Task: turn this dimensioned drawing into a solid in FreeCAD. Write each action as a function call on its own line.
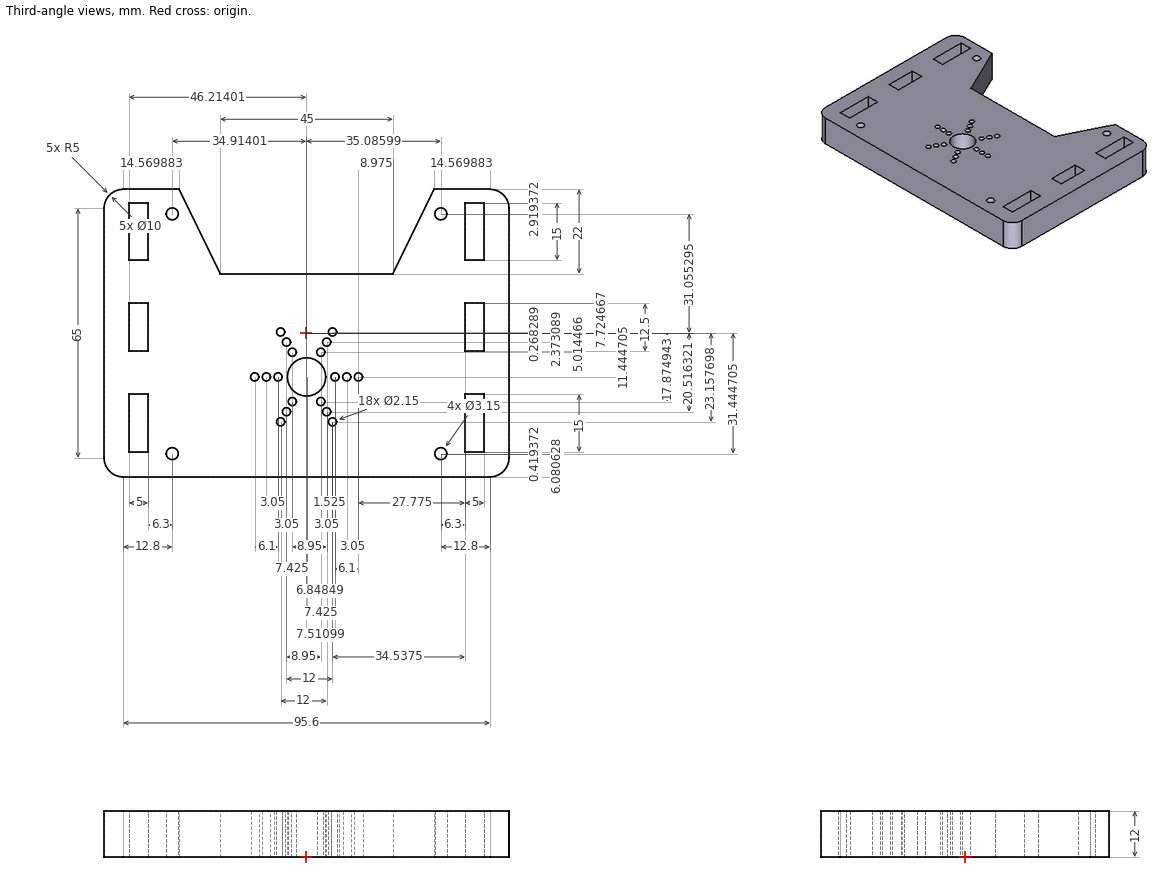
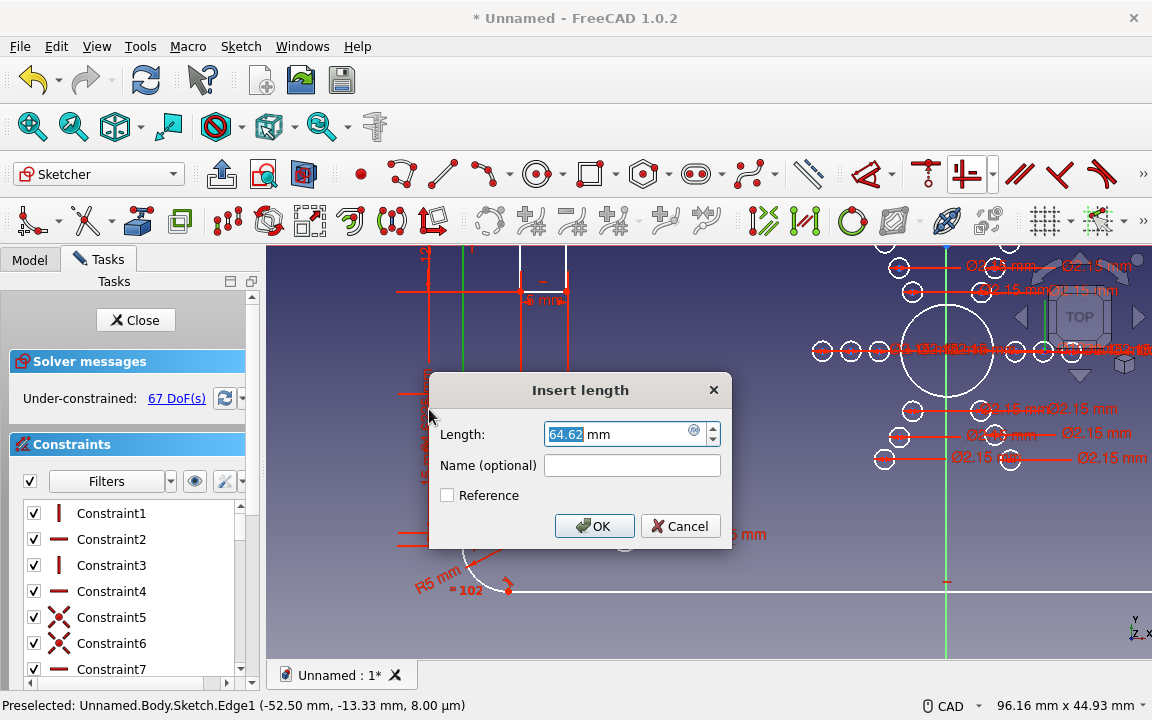
text(65)
key(Return)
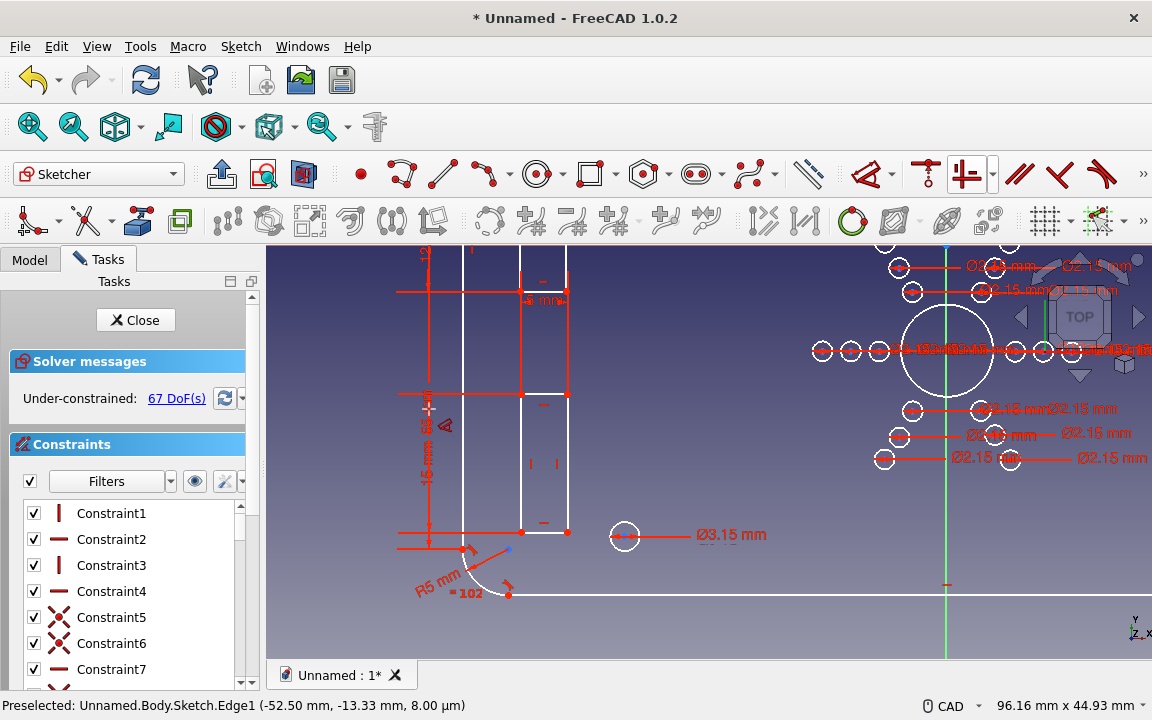
scroll(462, 572, down, 5)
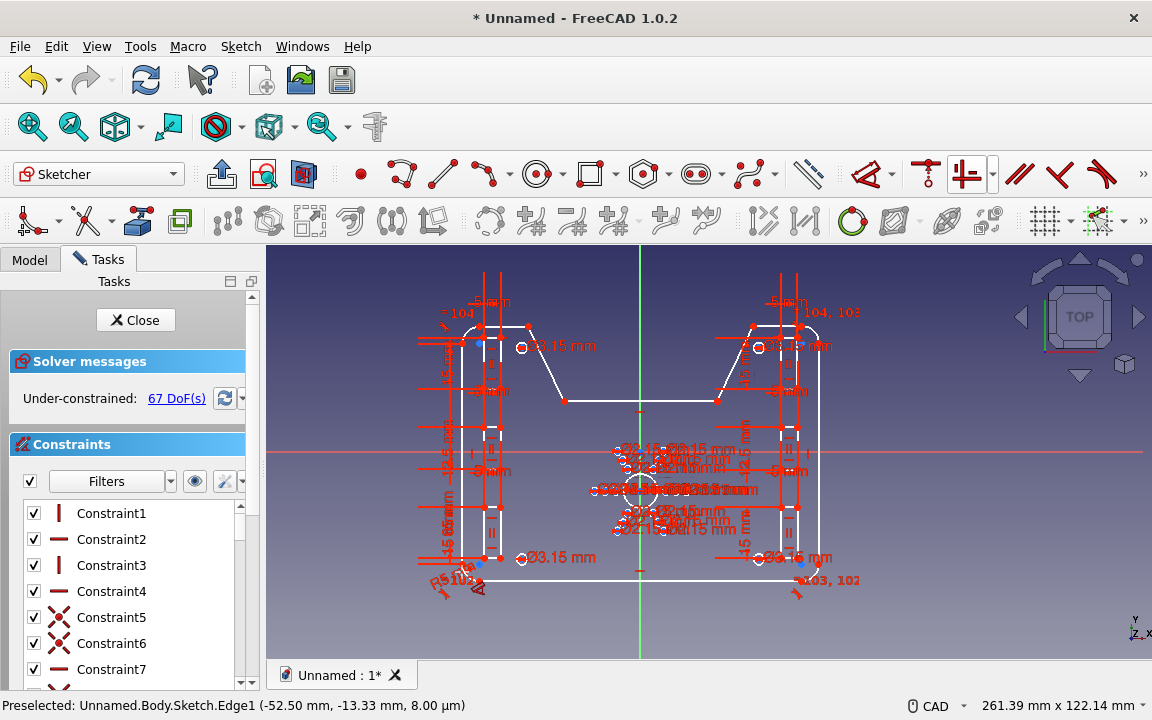
click(819, 498)
click(853, 403)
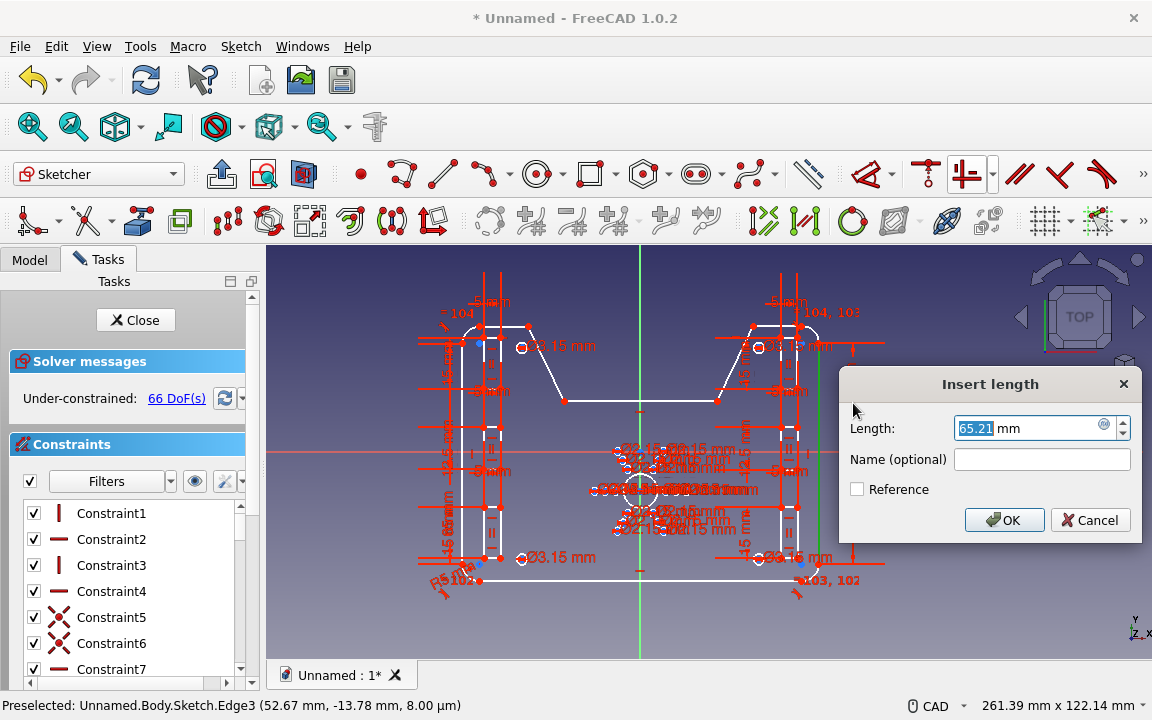
text(65)
key(Return)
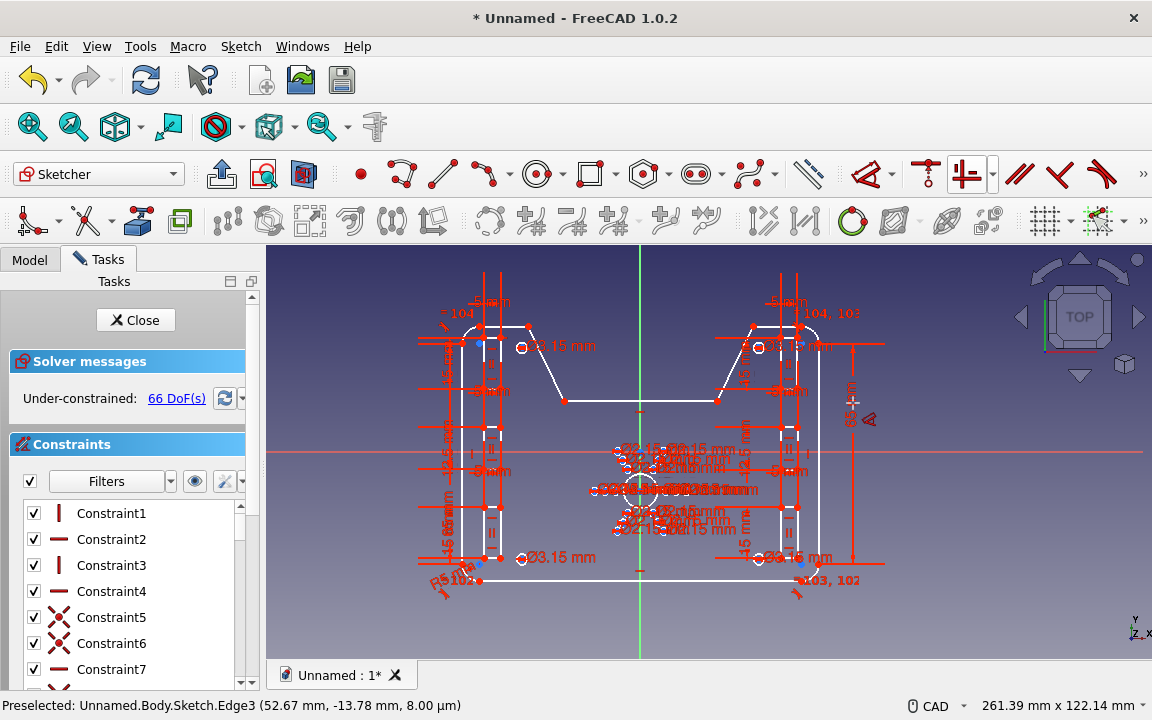
click(671, 401)
click(605, 367)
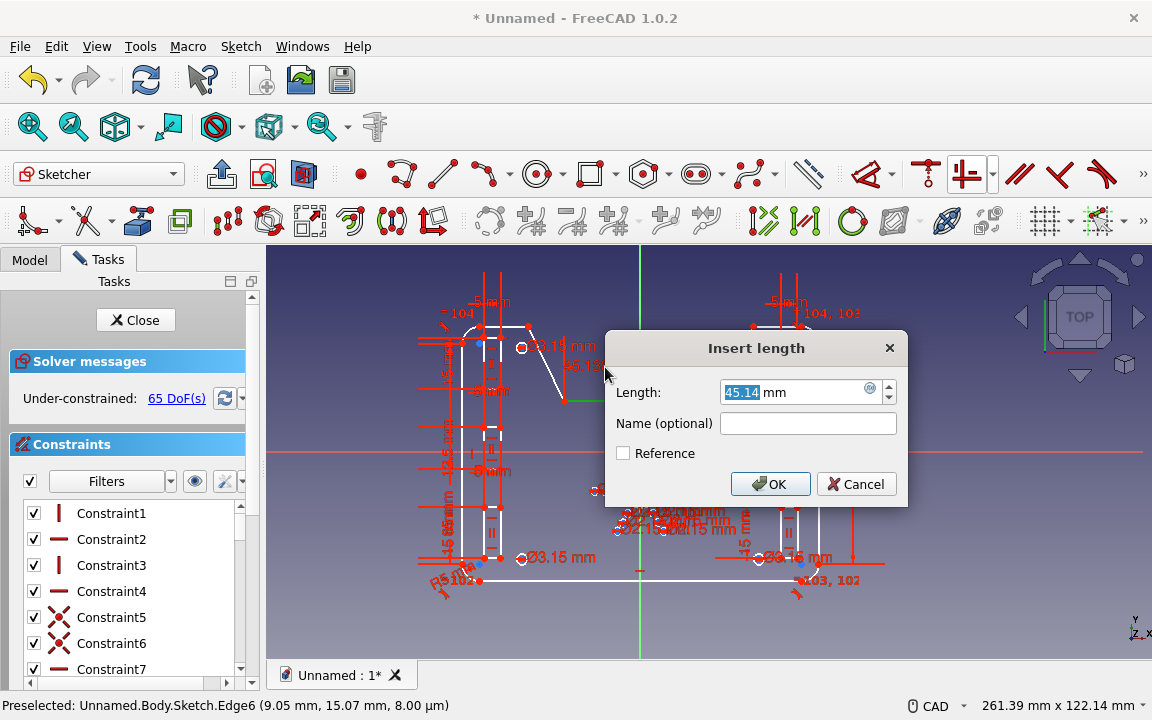
text(45)
key(Return)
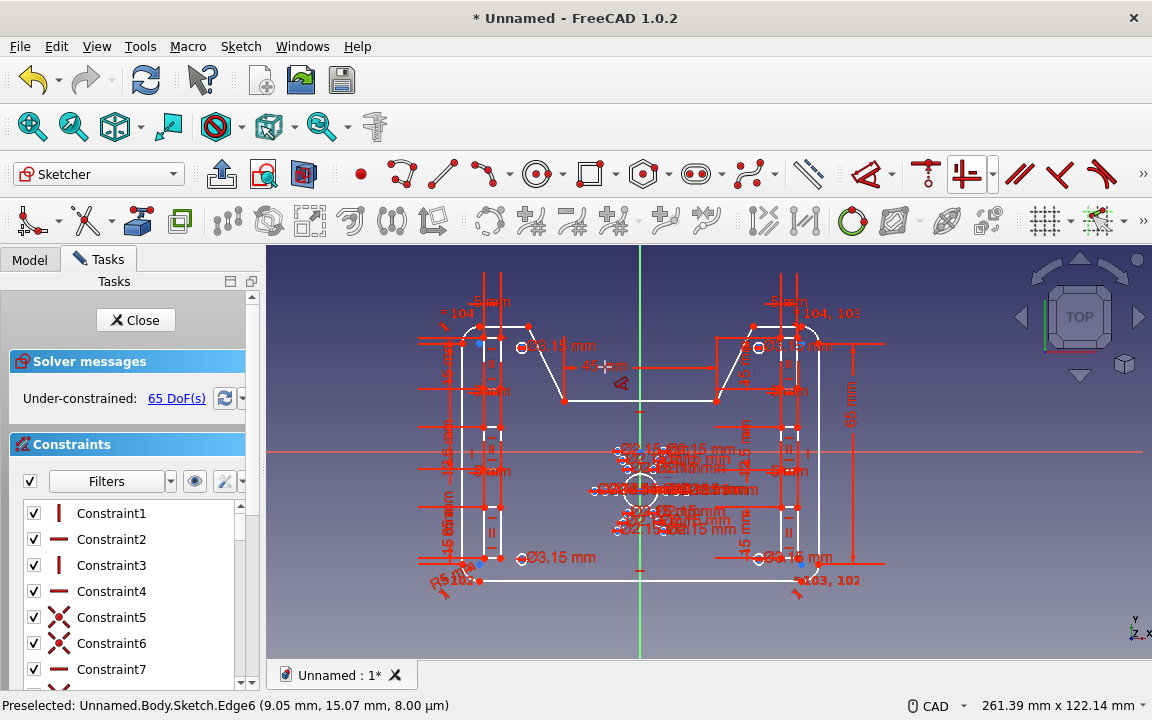
click(742, 349)
click(683, 364)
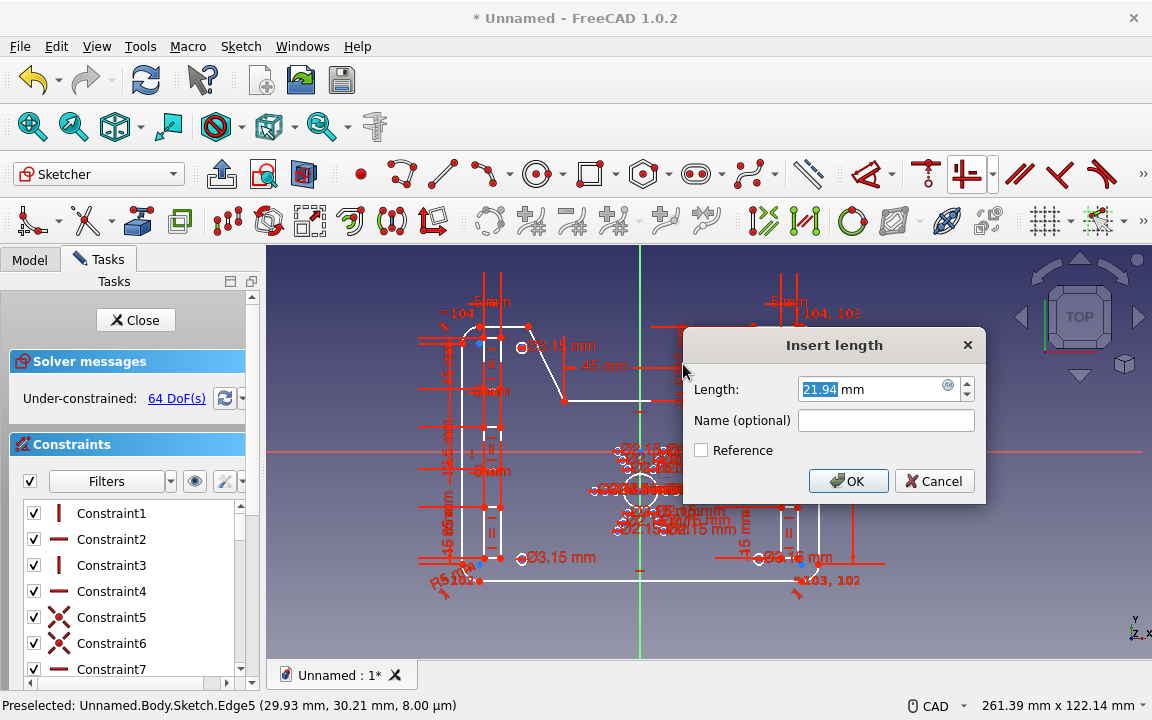
text(22)
key(Return)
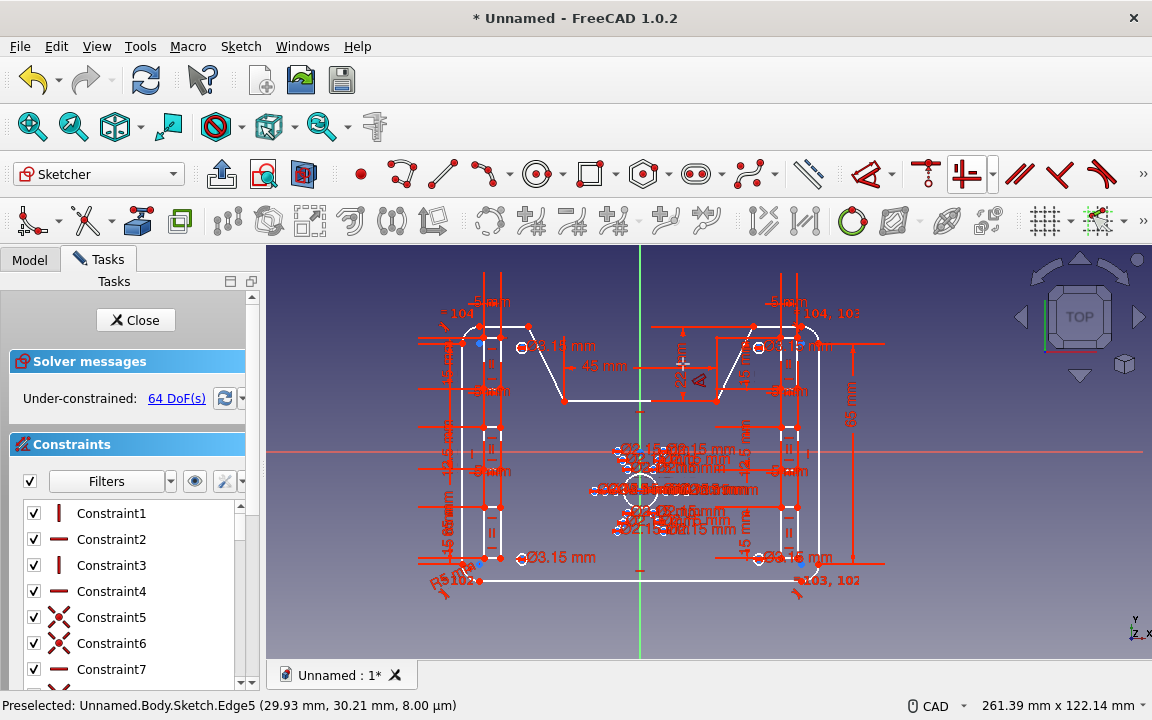
click(664, 531)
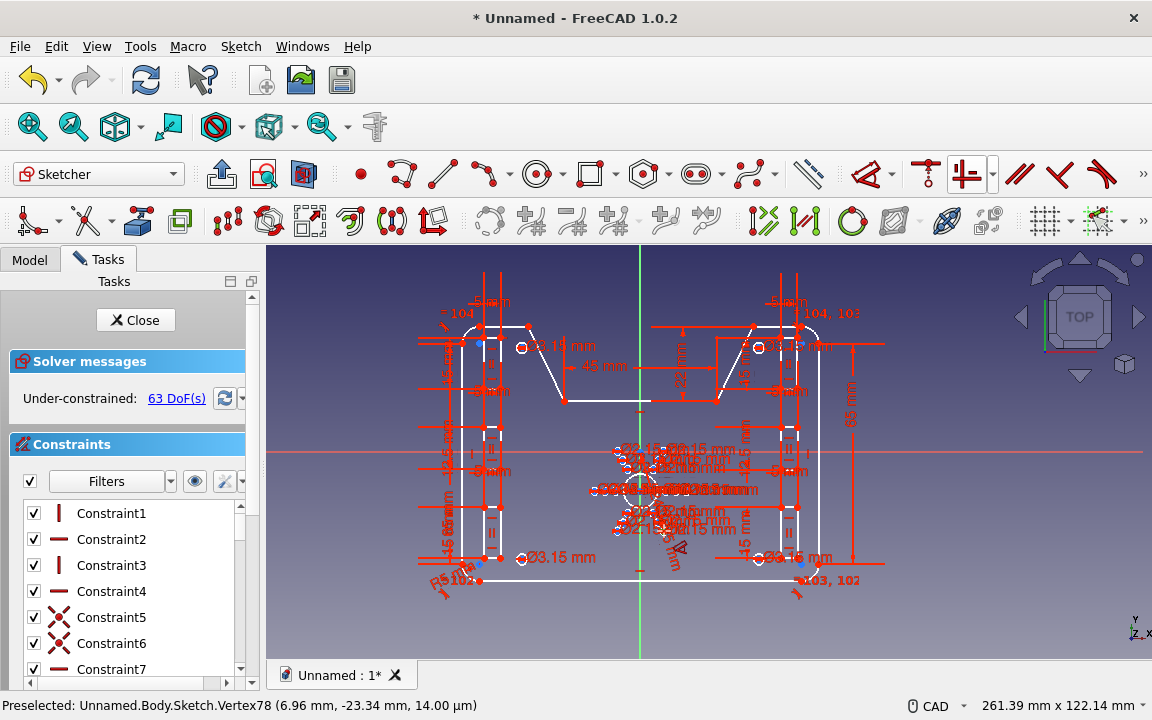
scroll(623, 523, up, 2)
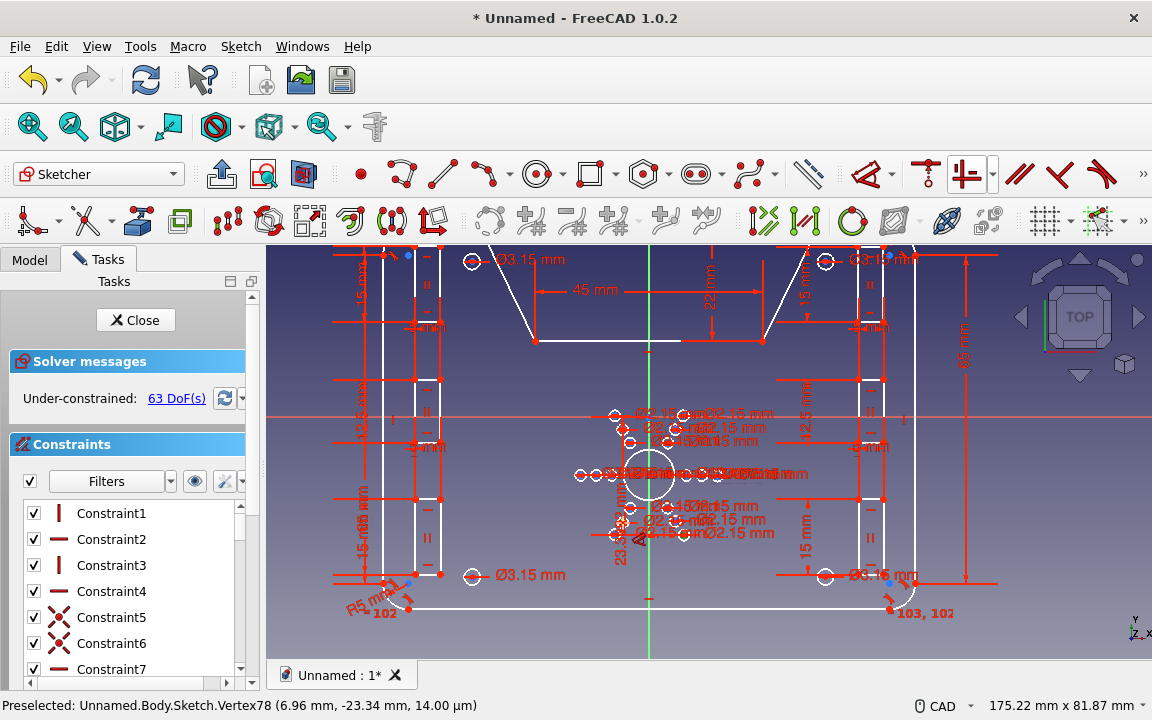
click(623, 523)
click(667, 569)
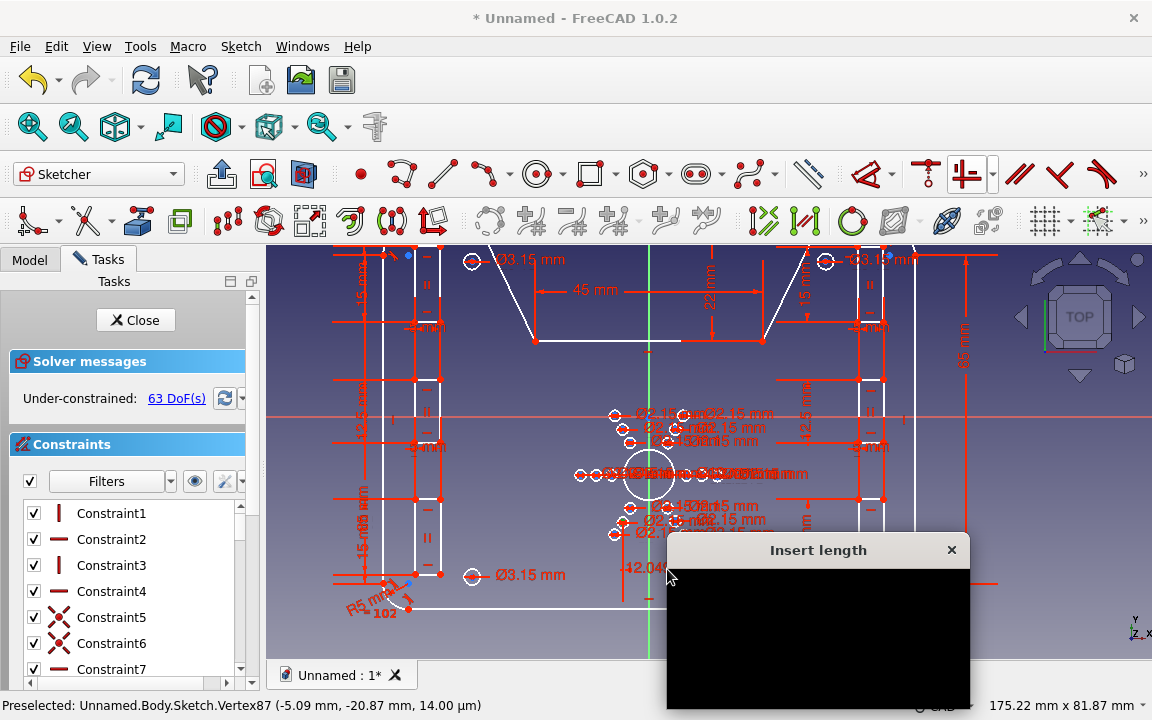
text(12)
key(Return)